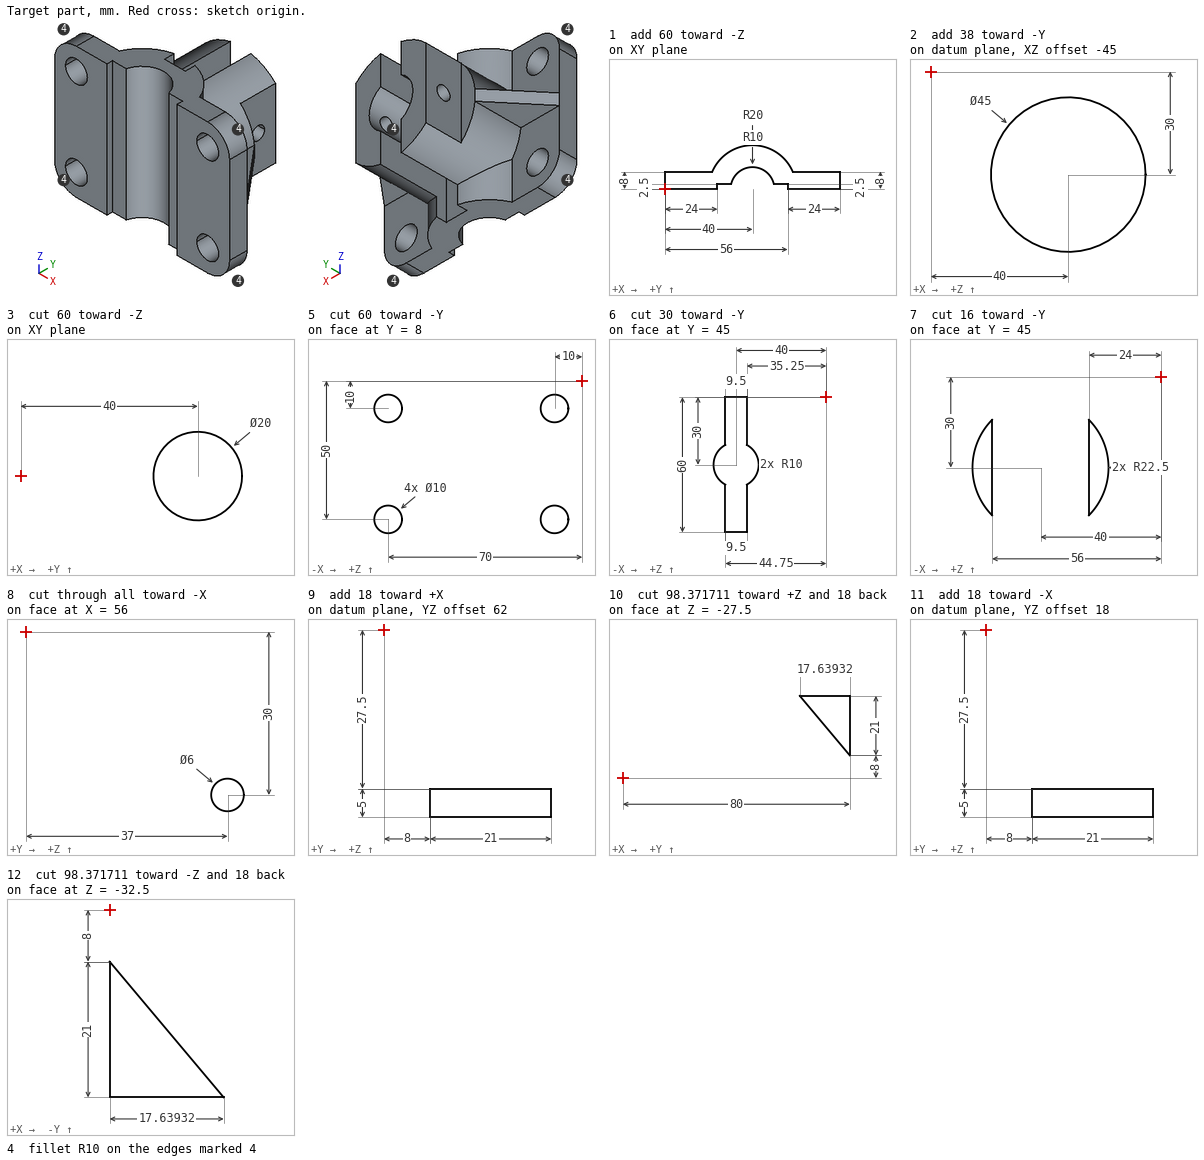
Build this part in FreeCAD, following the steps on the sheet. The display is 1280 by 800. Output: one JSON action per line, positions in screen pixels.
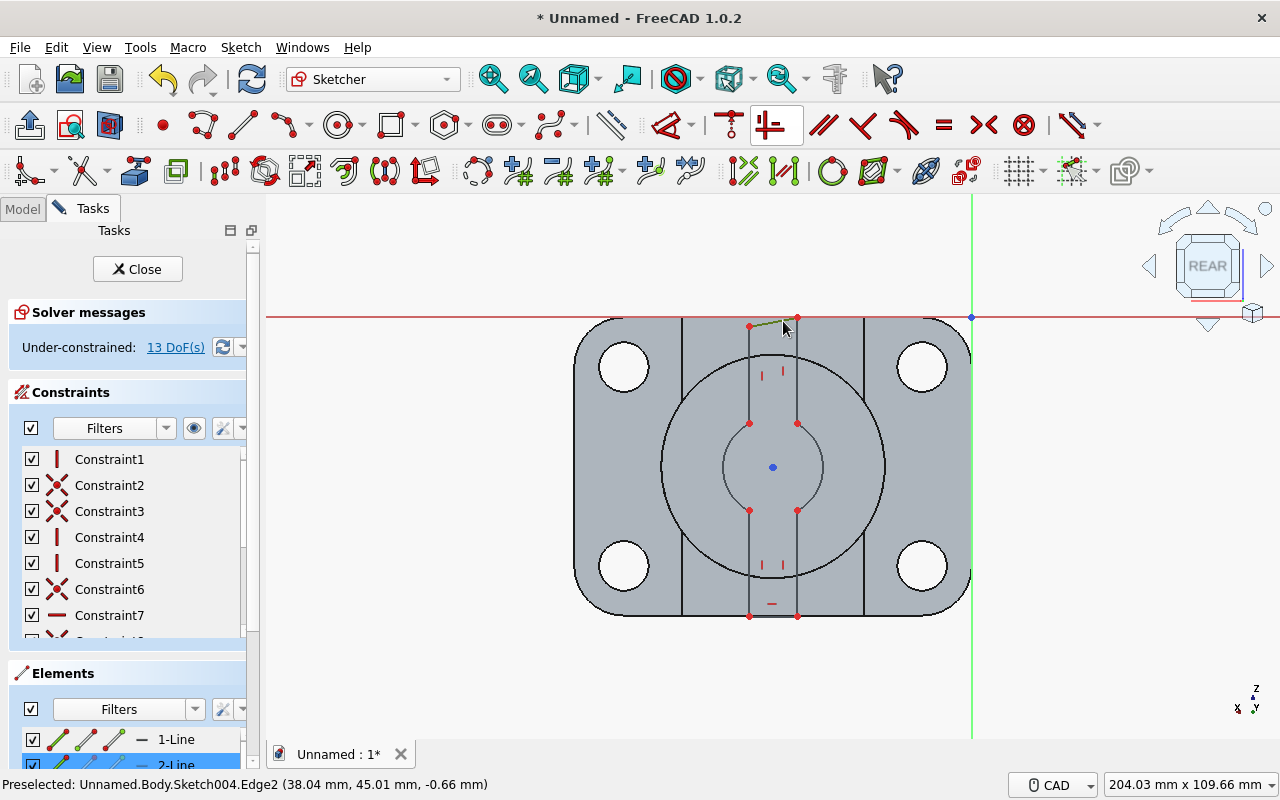
{"action": "left_click", "coordinate": [798, 126]}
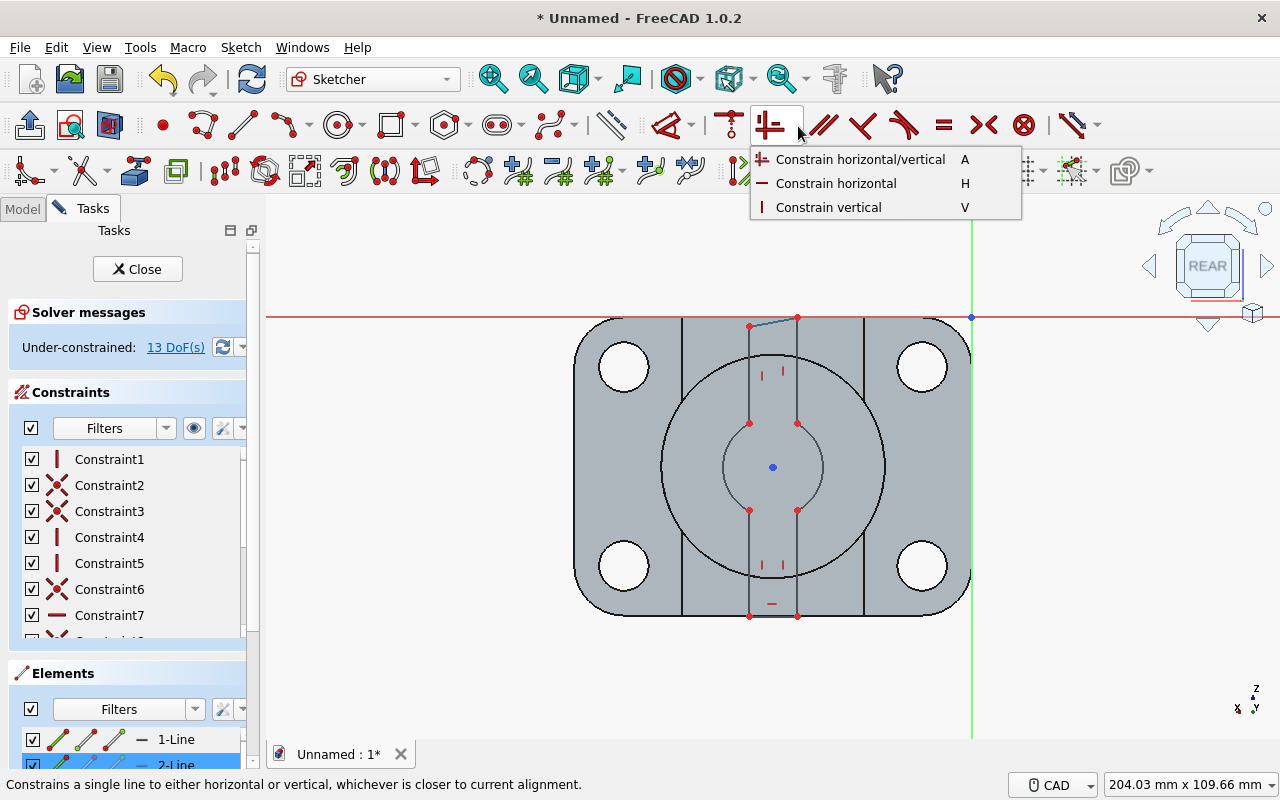
{"action": "left_click", "coordinate": [886, 183]}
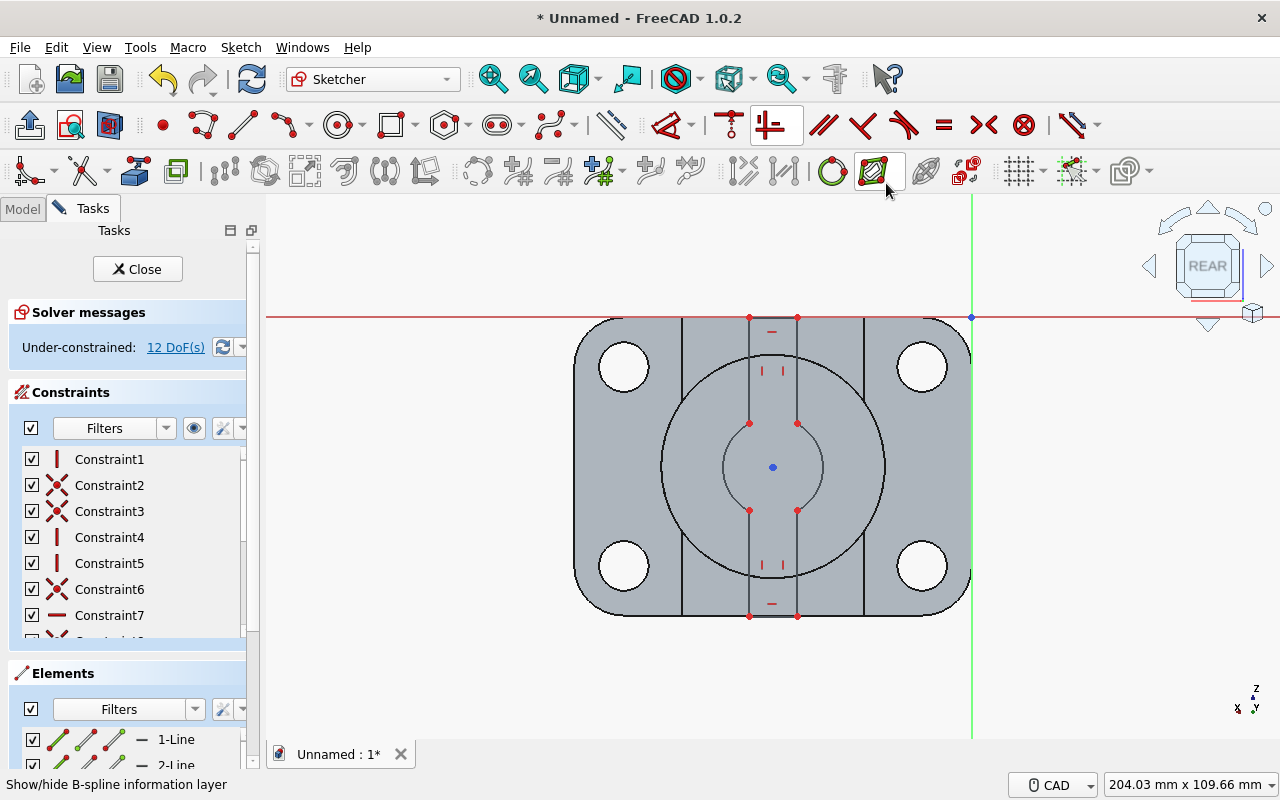
{"action": "left_click", "coordinate": [728, 447]}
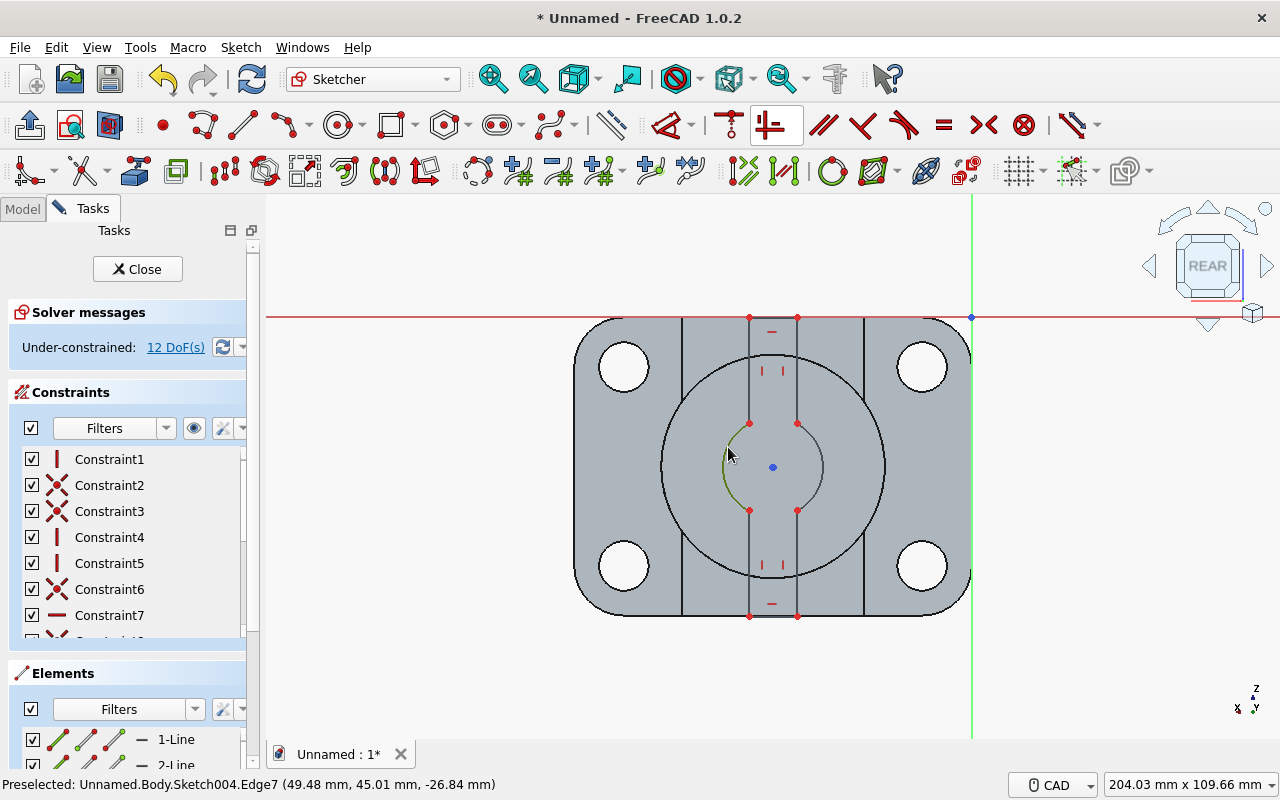
{"action": "left_click", "coordinate": [818, 488]}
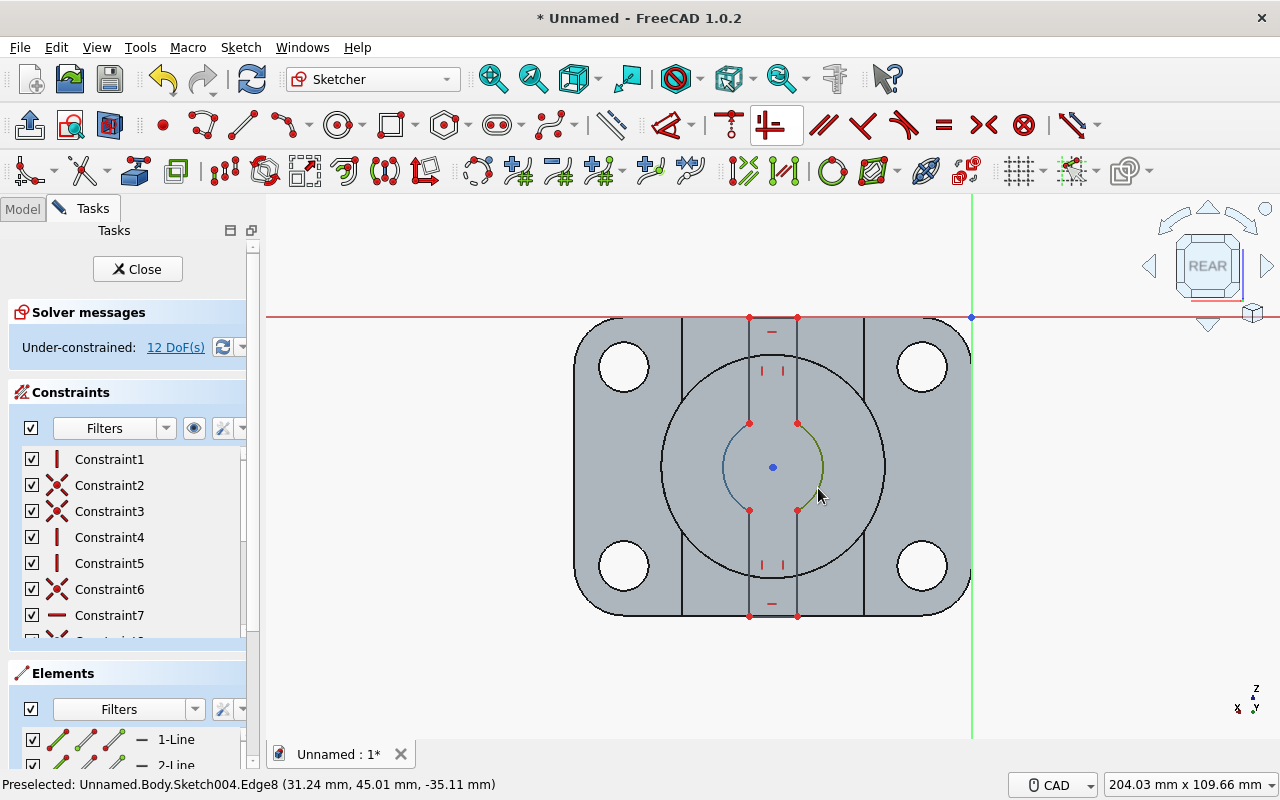
{"action": "left_click", "coordinate": [730, 126]}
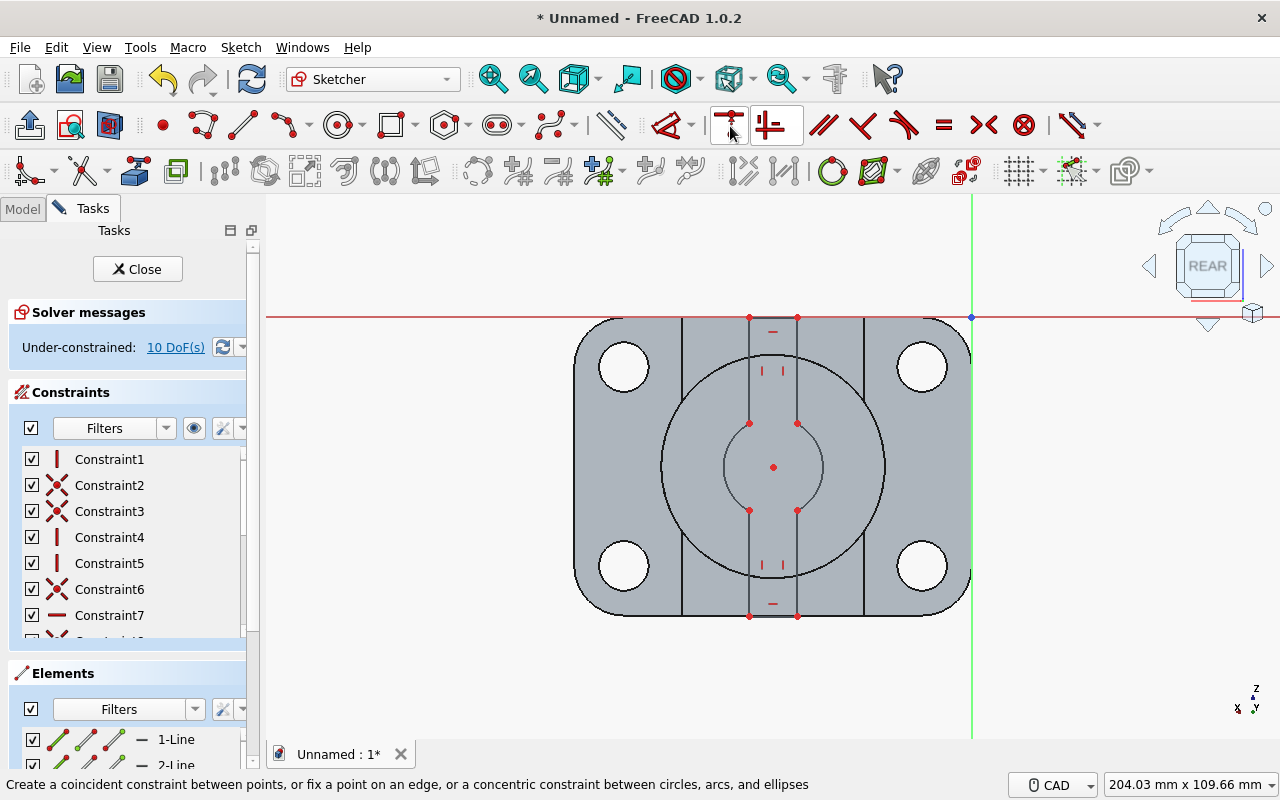
{"action": "left_click", "coordinate": [728, 447]}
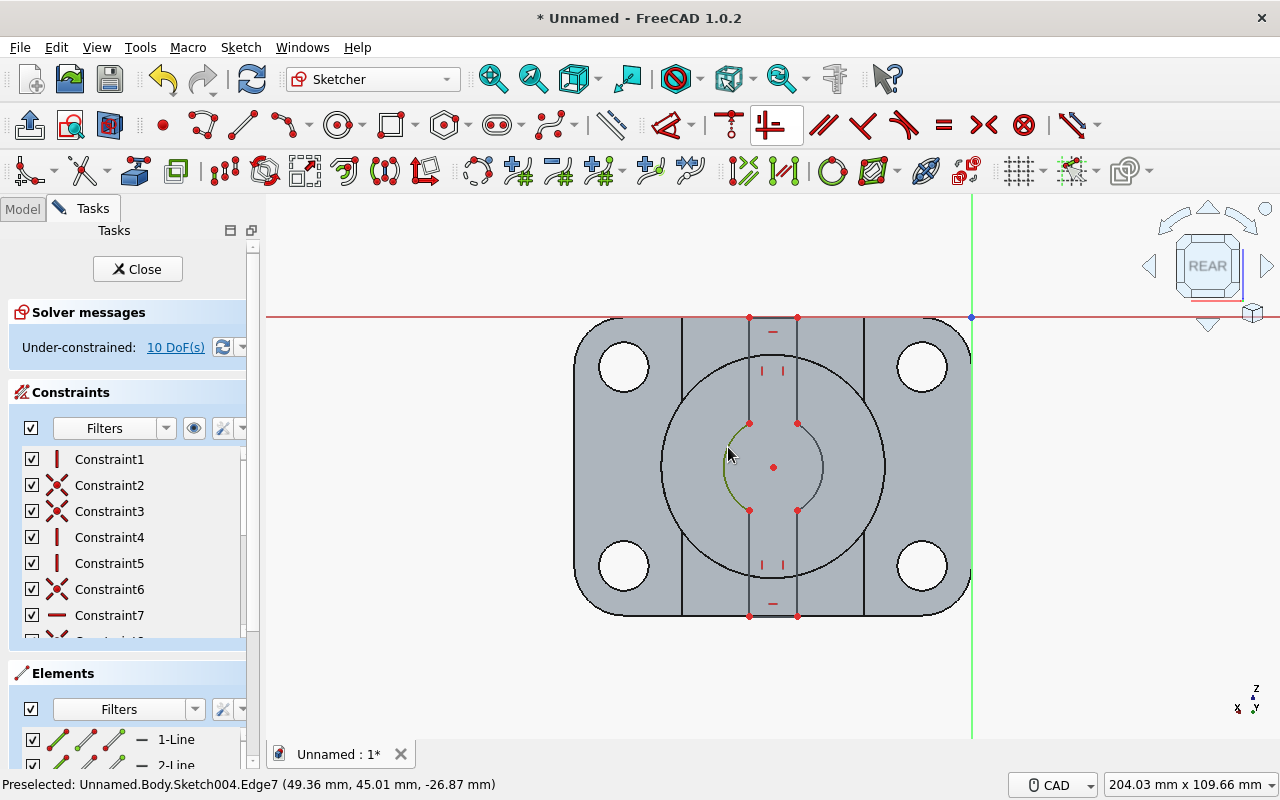
{"action": "left_click", "coordinate": [818, 488]}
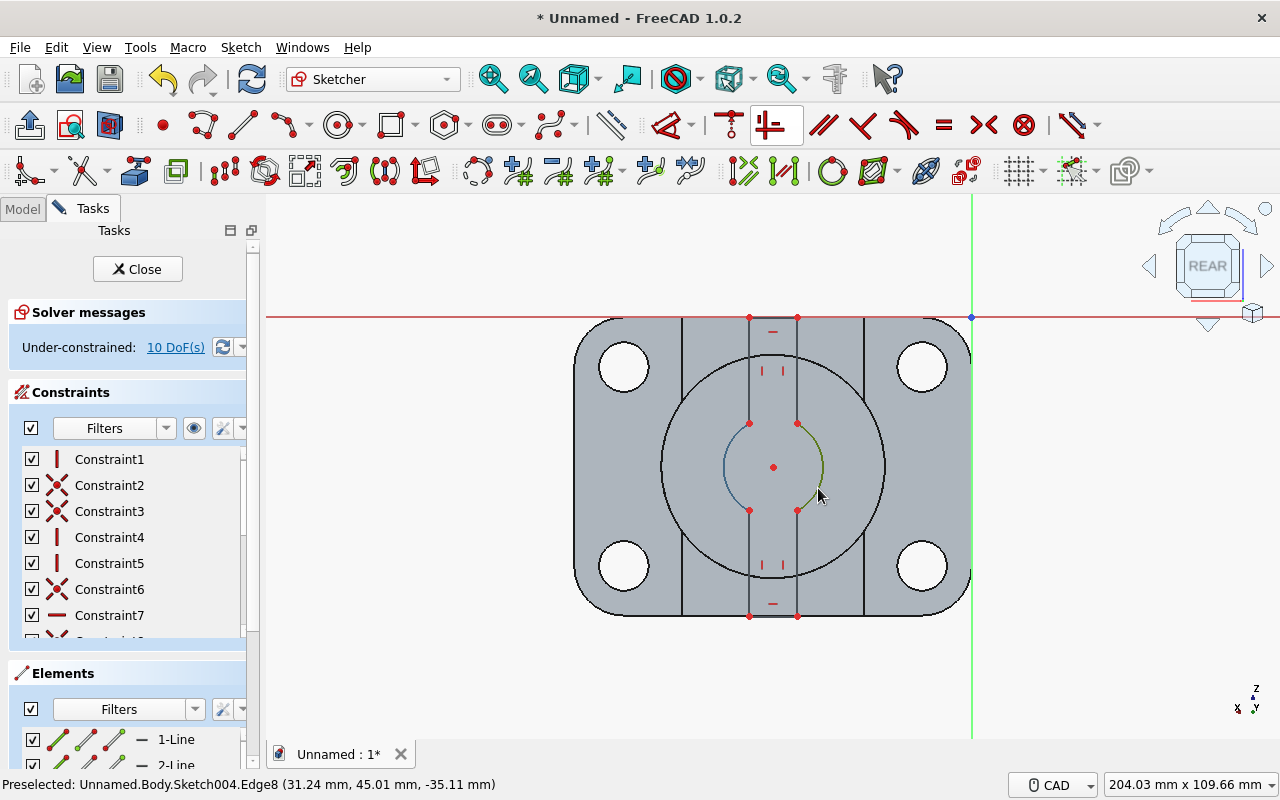
{"action": "left_click", "coordinate": [944, 126]}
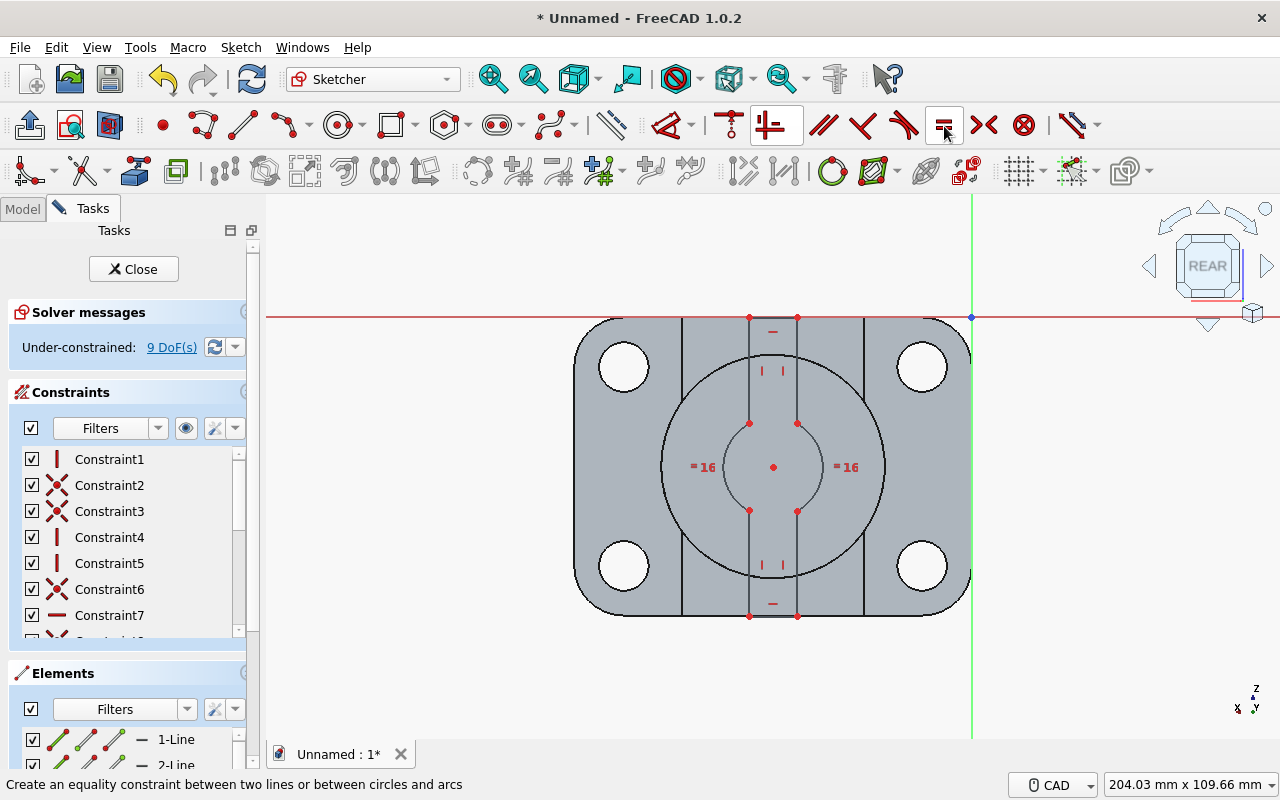
{"action": "left_click", "coordinate": [666, 126]}